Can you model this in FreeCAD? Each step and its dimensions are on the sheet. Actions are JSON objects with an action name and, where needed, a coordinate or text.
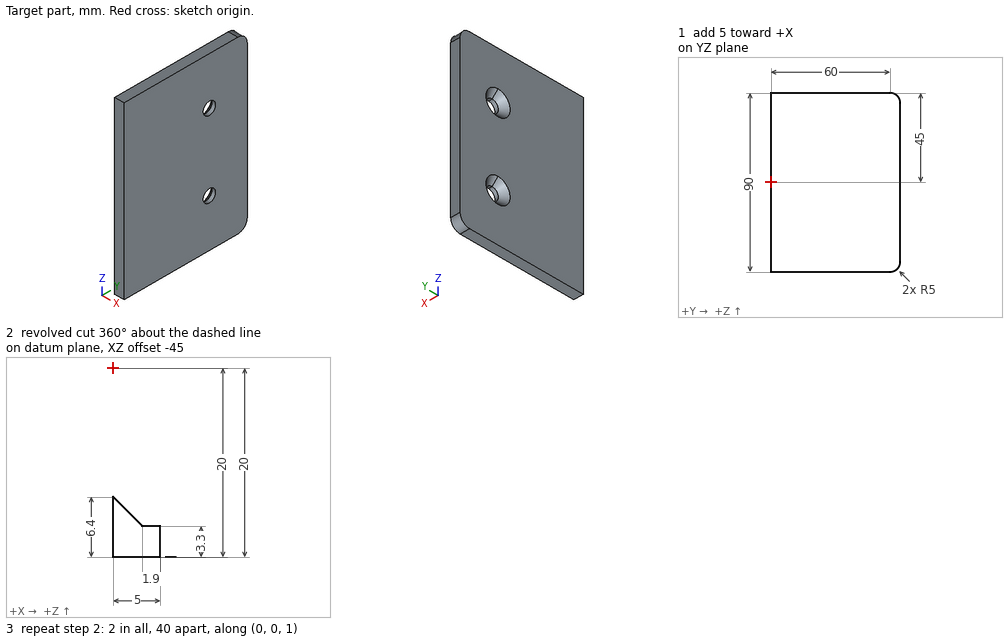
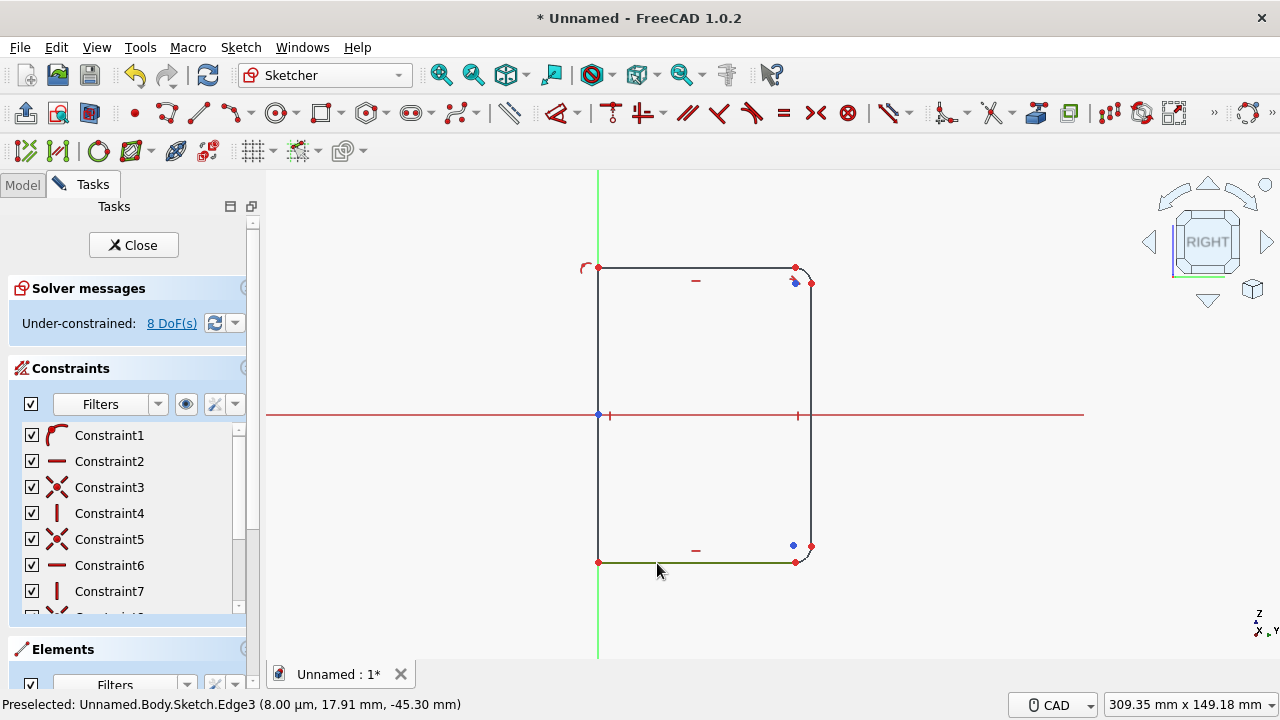
{"action": "left_click", "coordinate": [806, 558]}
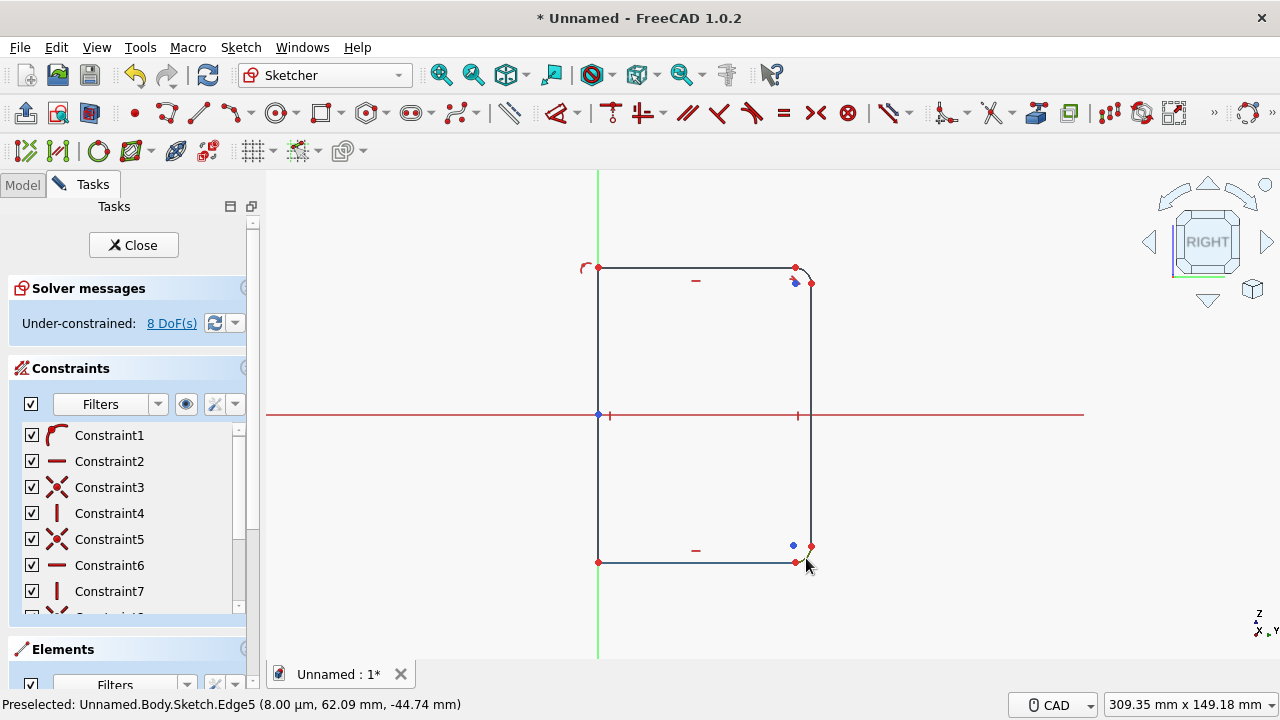
{"action": "left_click", "coordinate": [752, 114]}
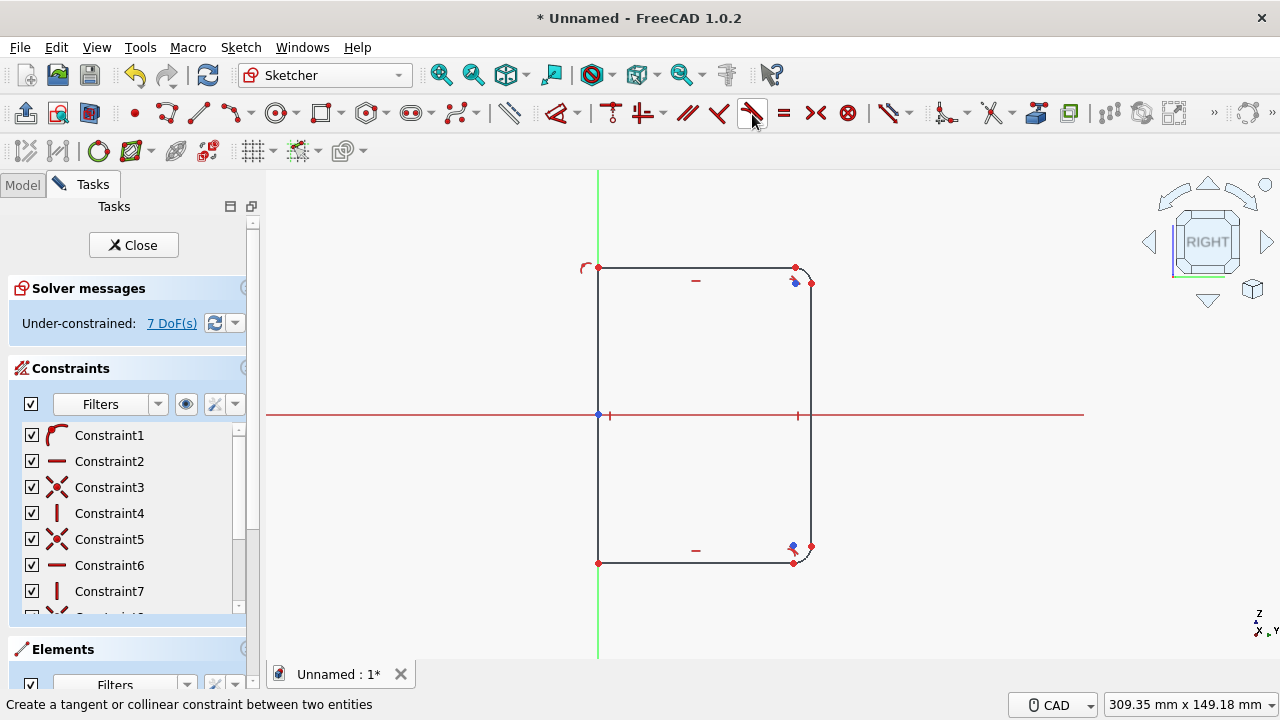
{"action": "left_click", "coordinate": [811, 468]}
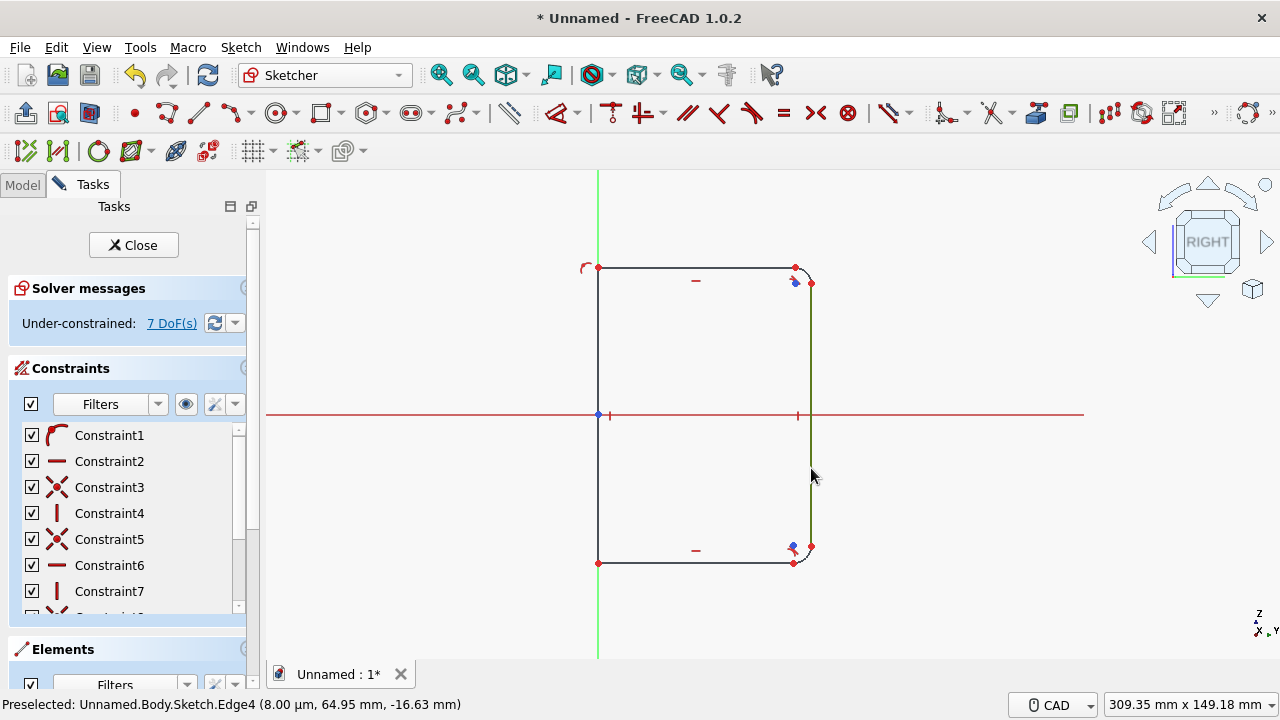
{"action": "left_click", "coordinate": [806, 558]}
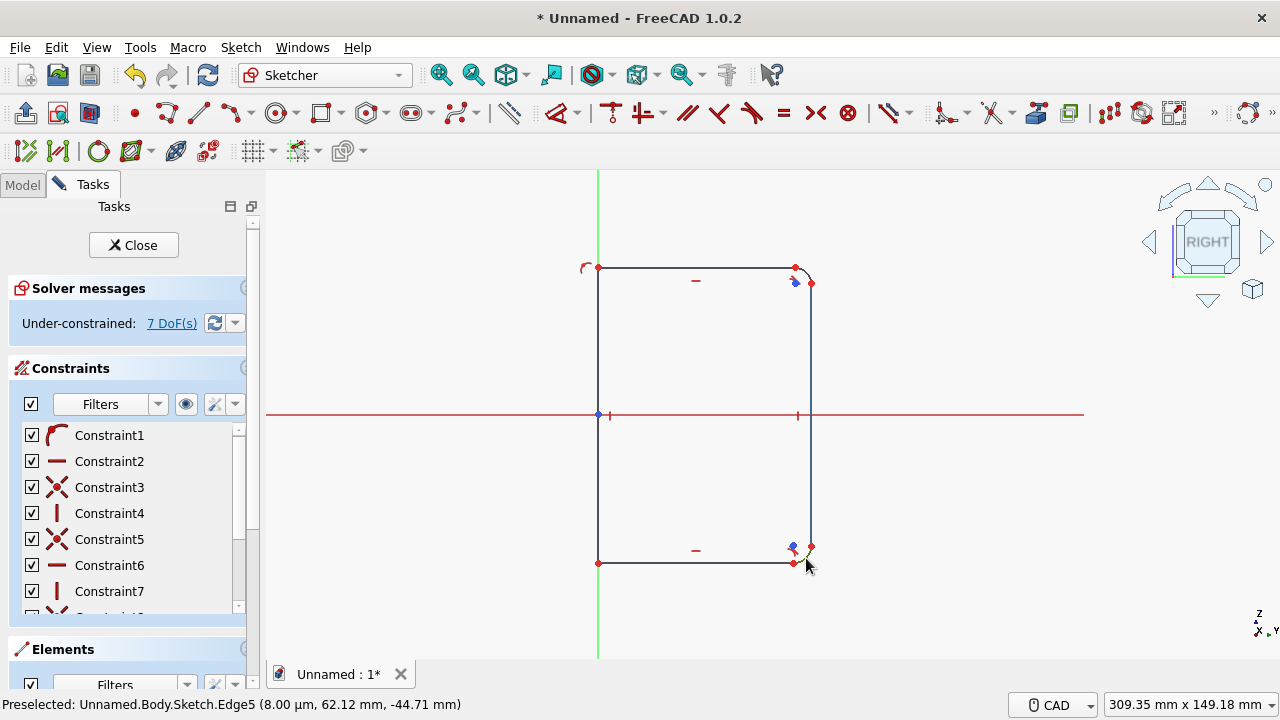
{"action": "left_click", "coordinate": [752, 114]}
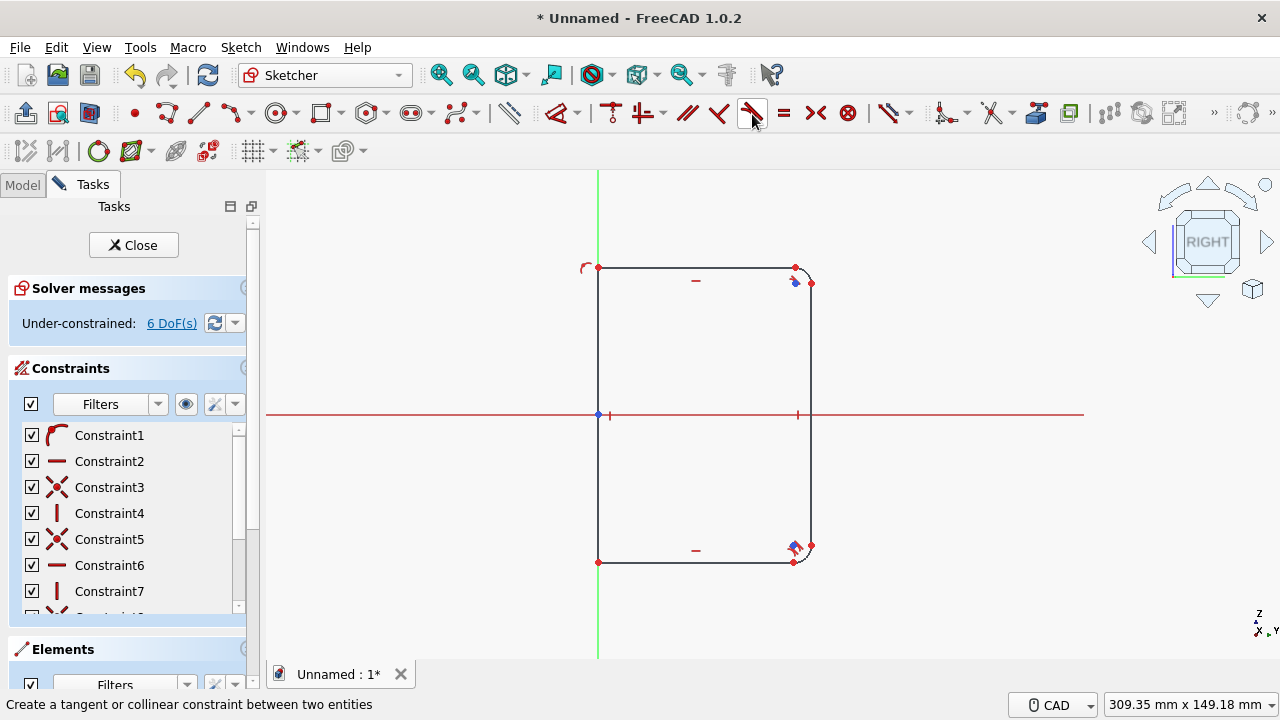
{"action": "left_click", "coordinate": [811, 467]}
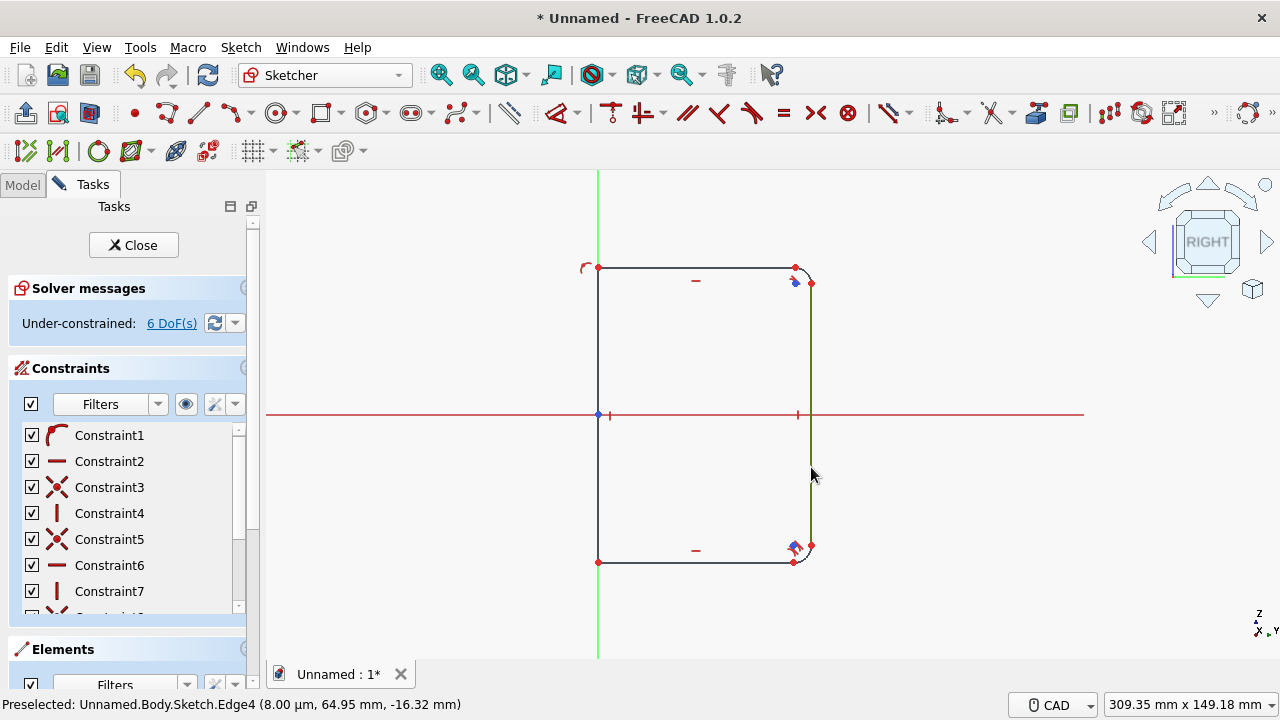
{"action": "left_click", "coordinate": [807, 273]}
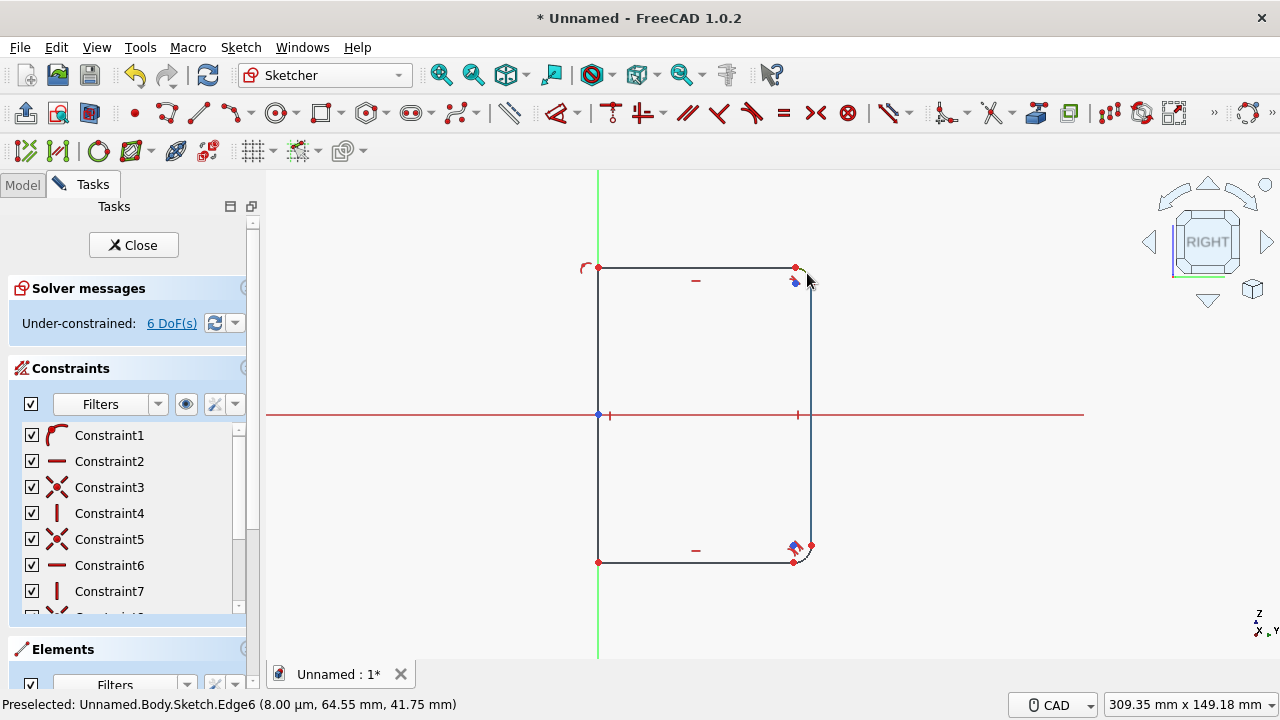
{"action": "left_click", "coordinate": [752, 114]}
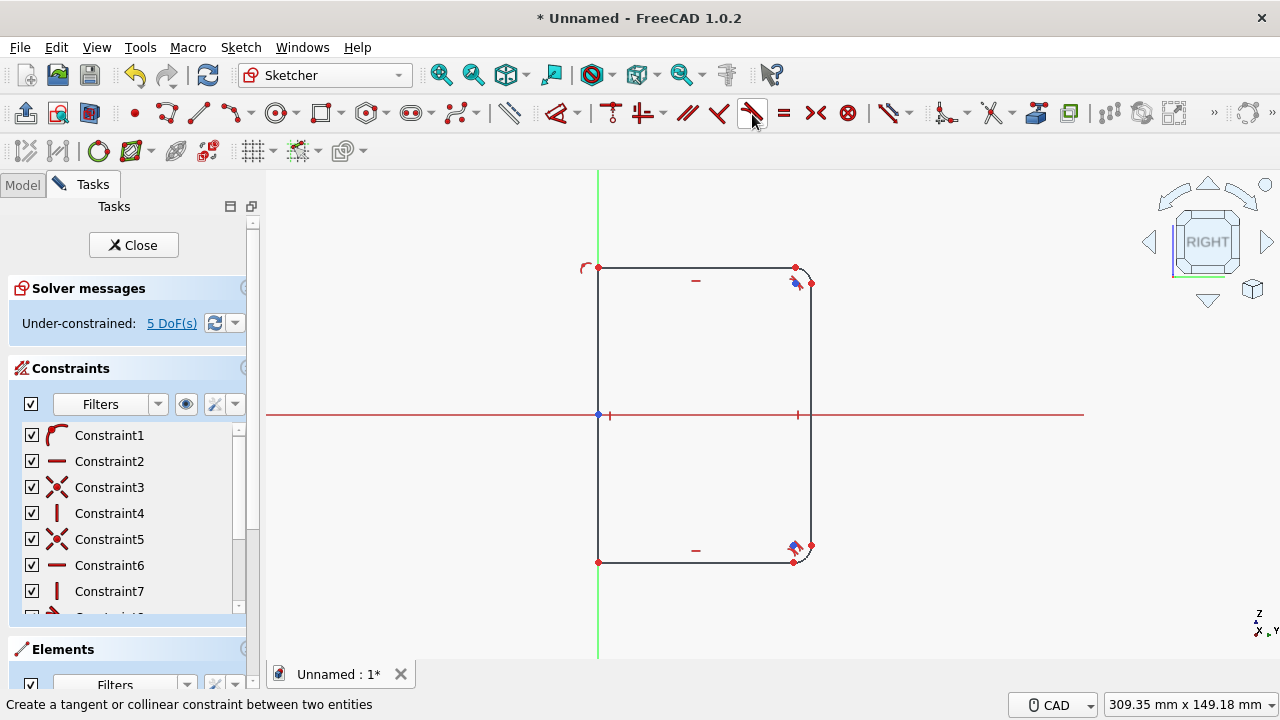
{"action": "left_click", "coordinate": [806, 558]}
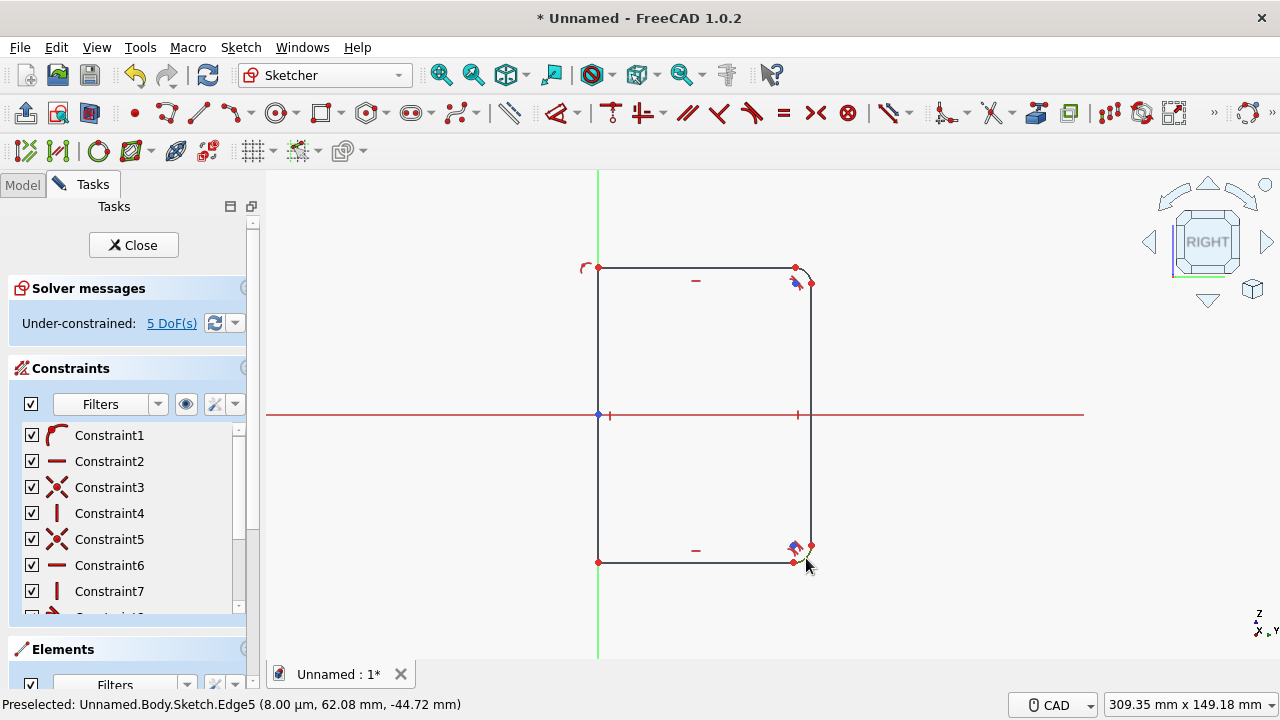
{"action": "left_click", "coordinate": [807, 273]}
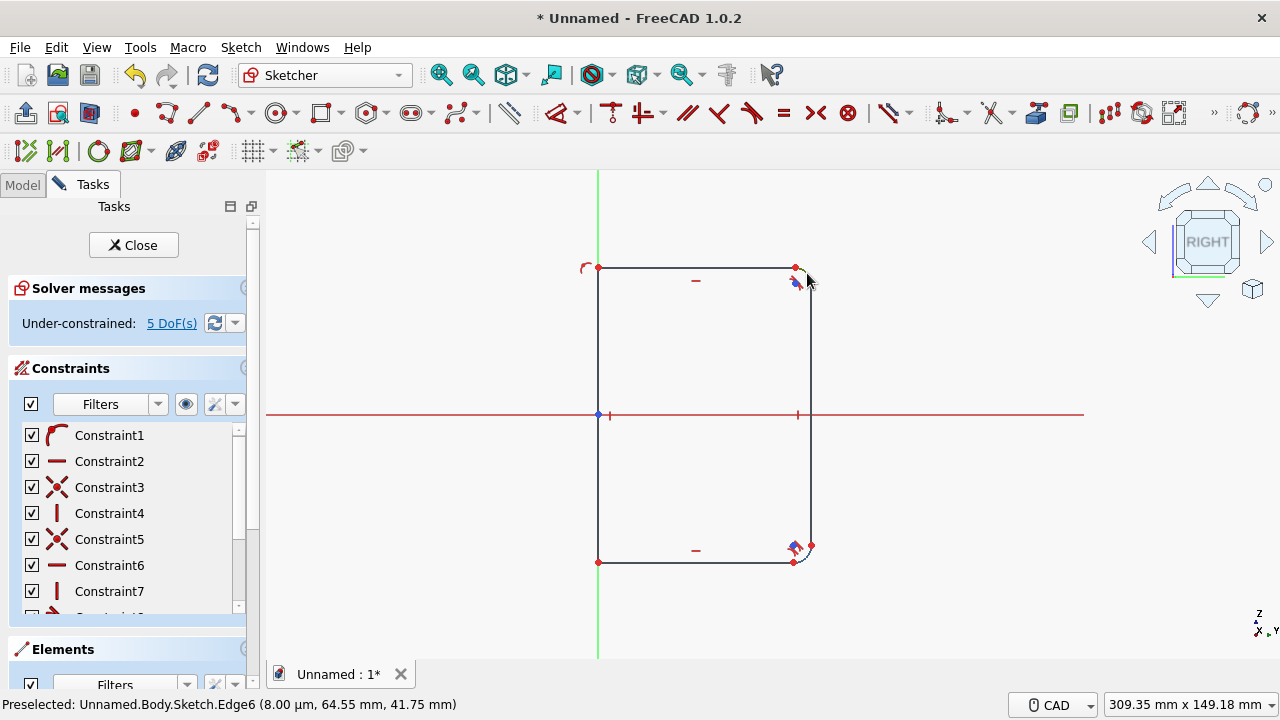
{"action": "left_click", "coordinate": [784, 114]}